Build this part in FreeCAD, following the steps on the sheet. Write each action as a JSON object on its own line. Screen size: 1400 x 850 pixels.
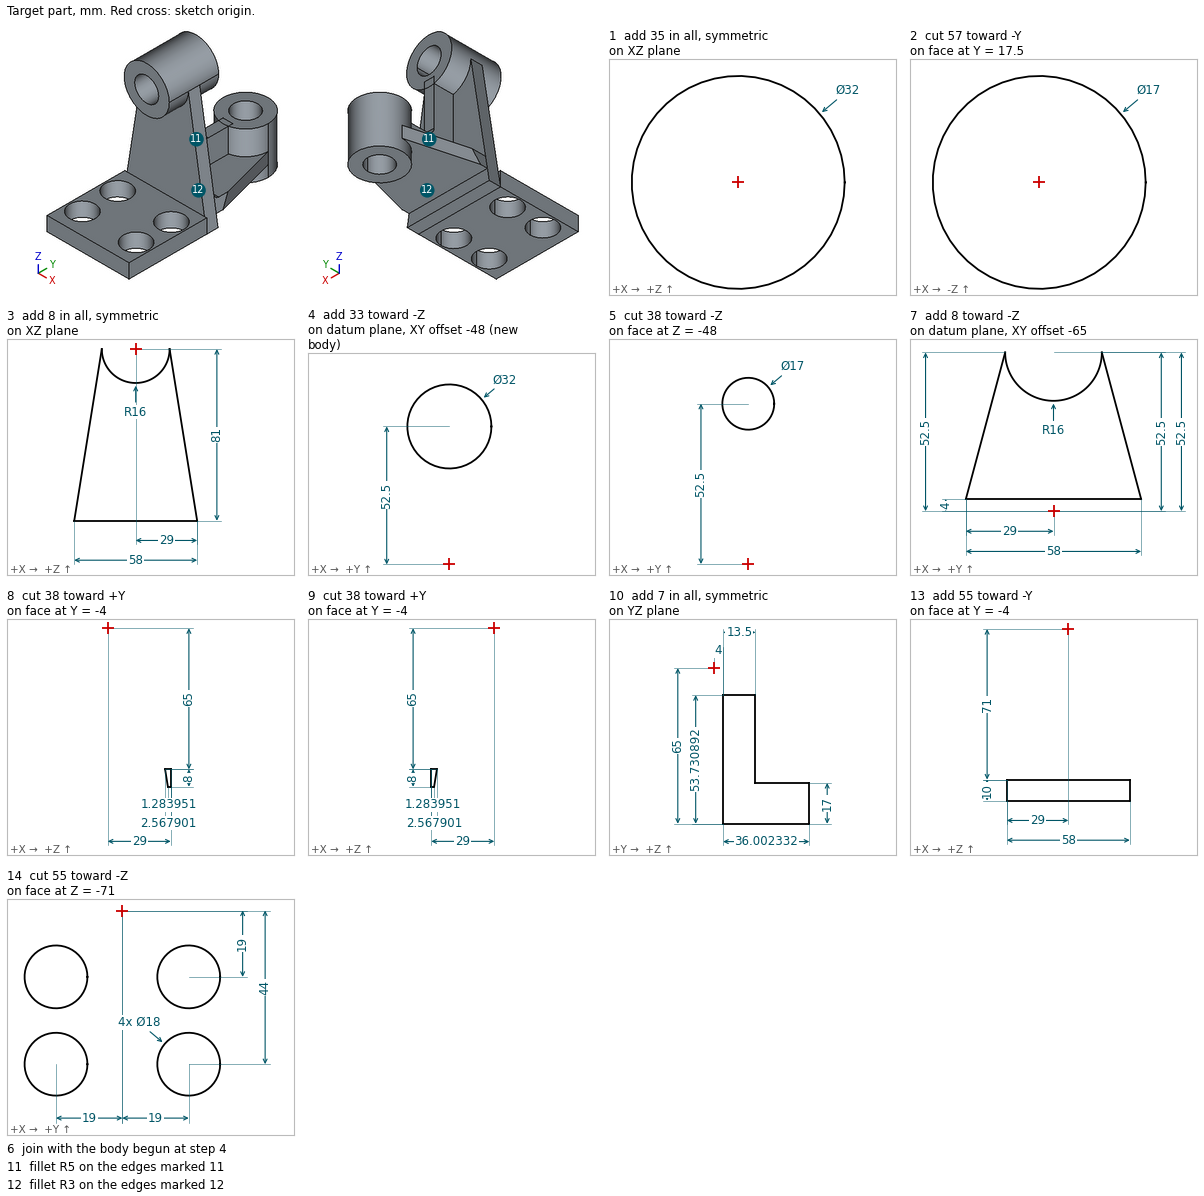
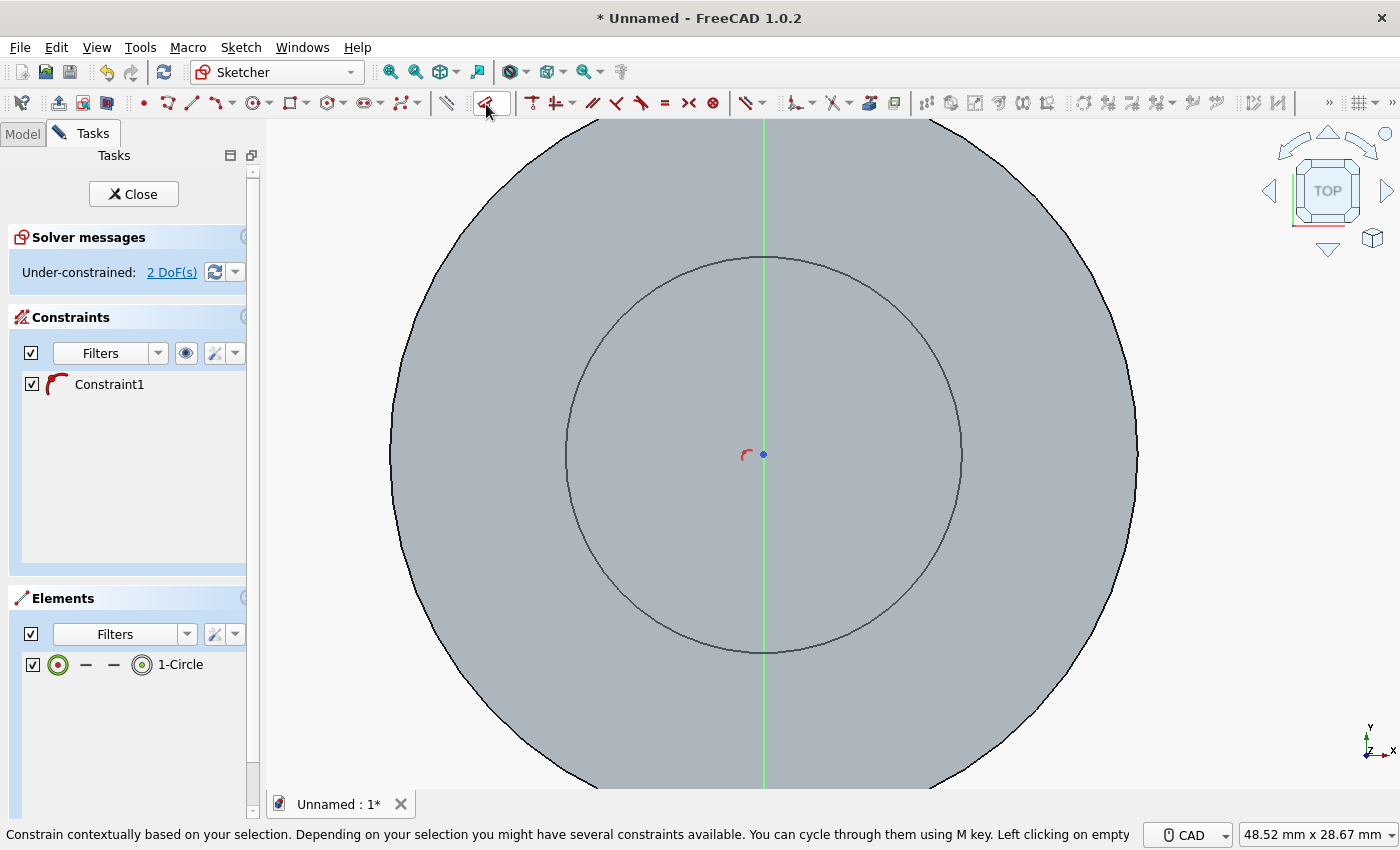
{"action": "left_click", "coordinate": [903, 314]}
{"action": "left_click", "coordinate": [925, 291]}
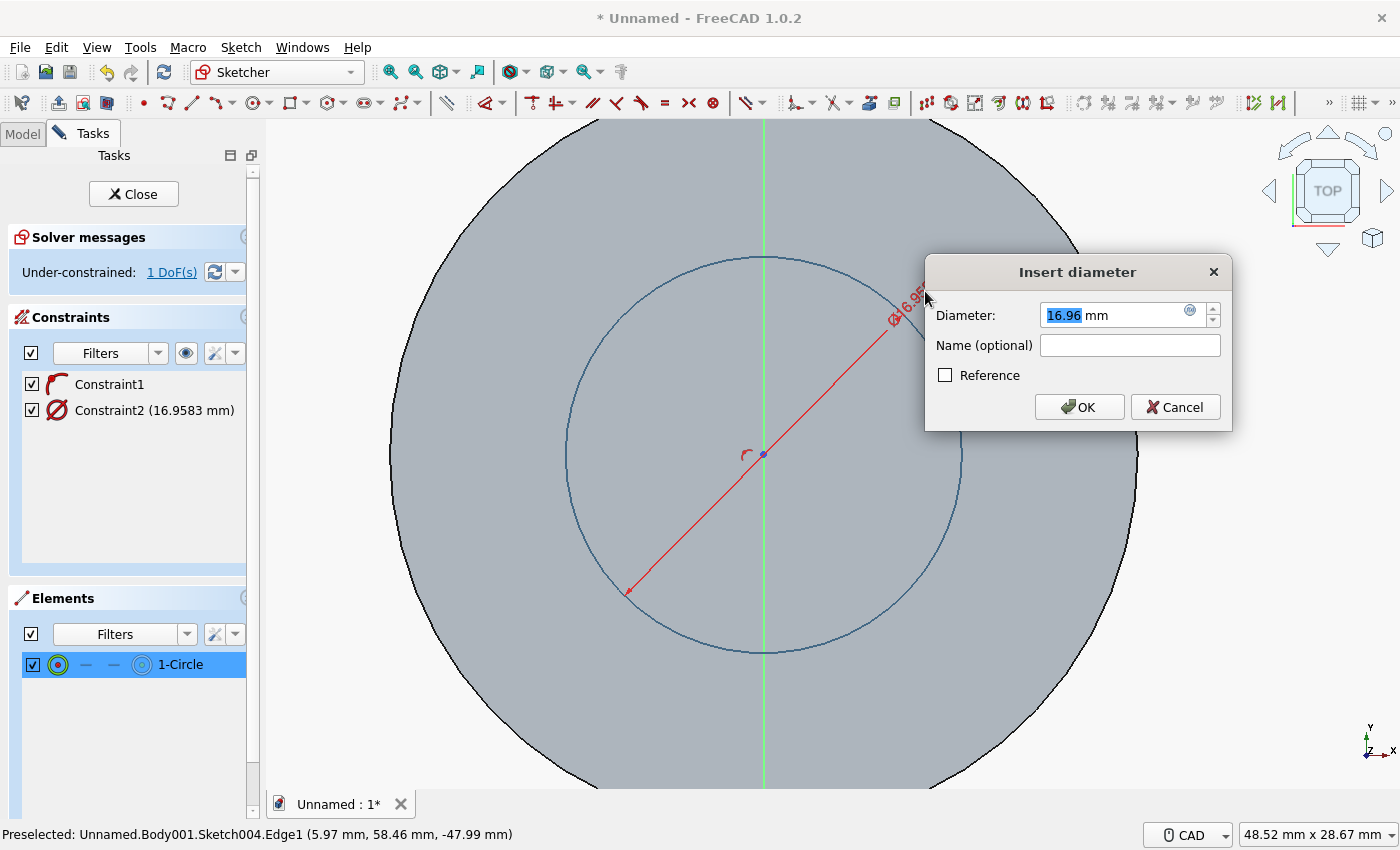
{"action": "type", "text": "17"}
{"action": "key", "text": "Return"}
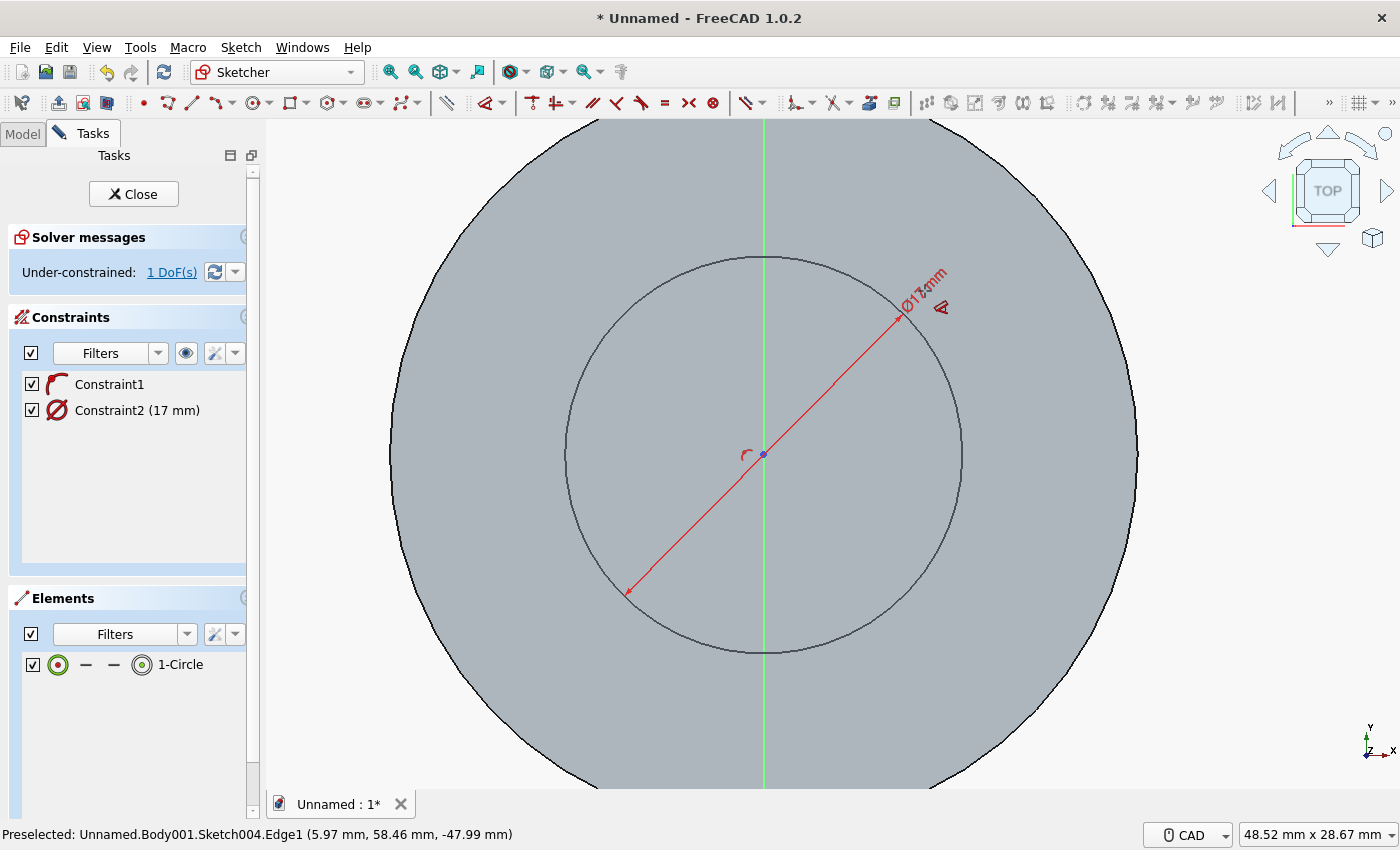
{"action": "left_click", "coordinate": [764, 455]}
{"action": "left_click", "coordinate": [798, 608]}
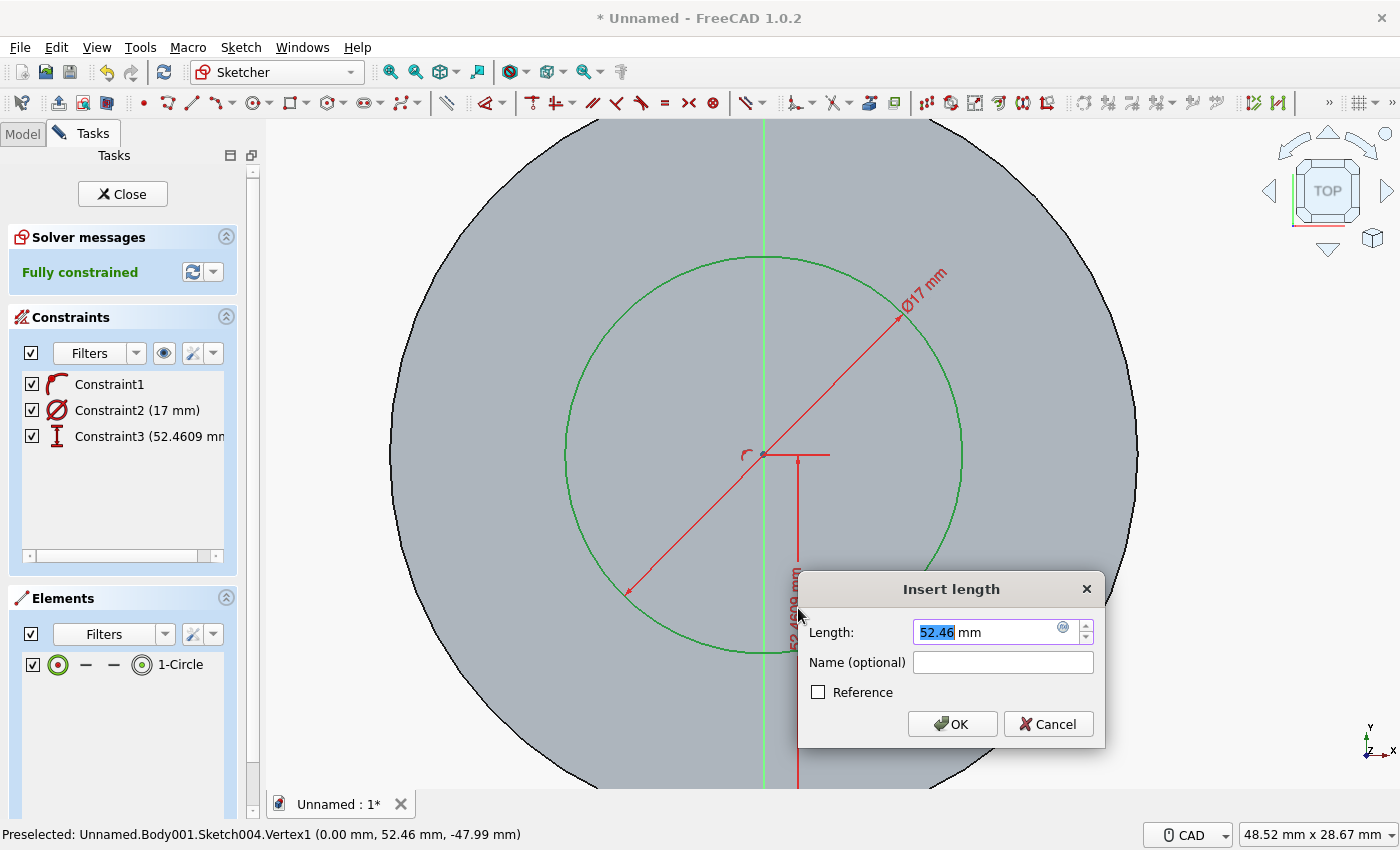
{"action": "type", "text": "52.5"}
{"action": "key", "text": "Return"}
{"action": "key", "text": "Escape"}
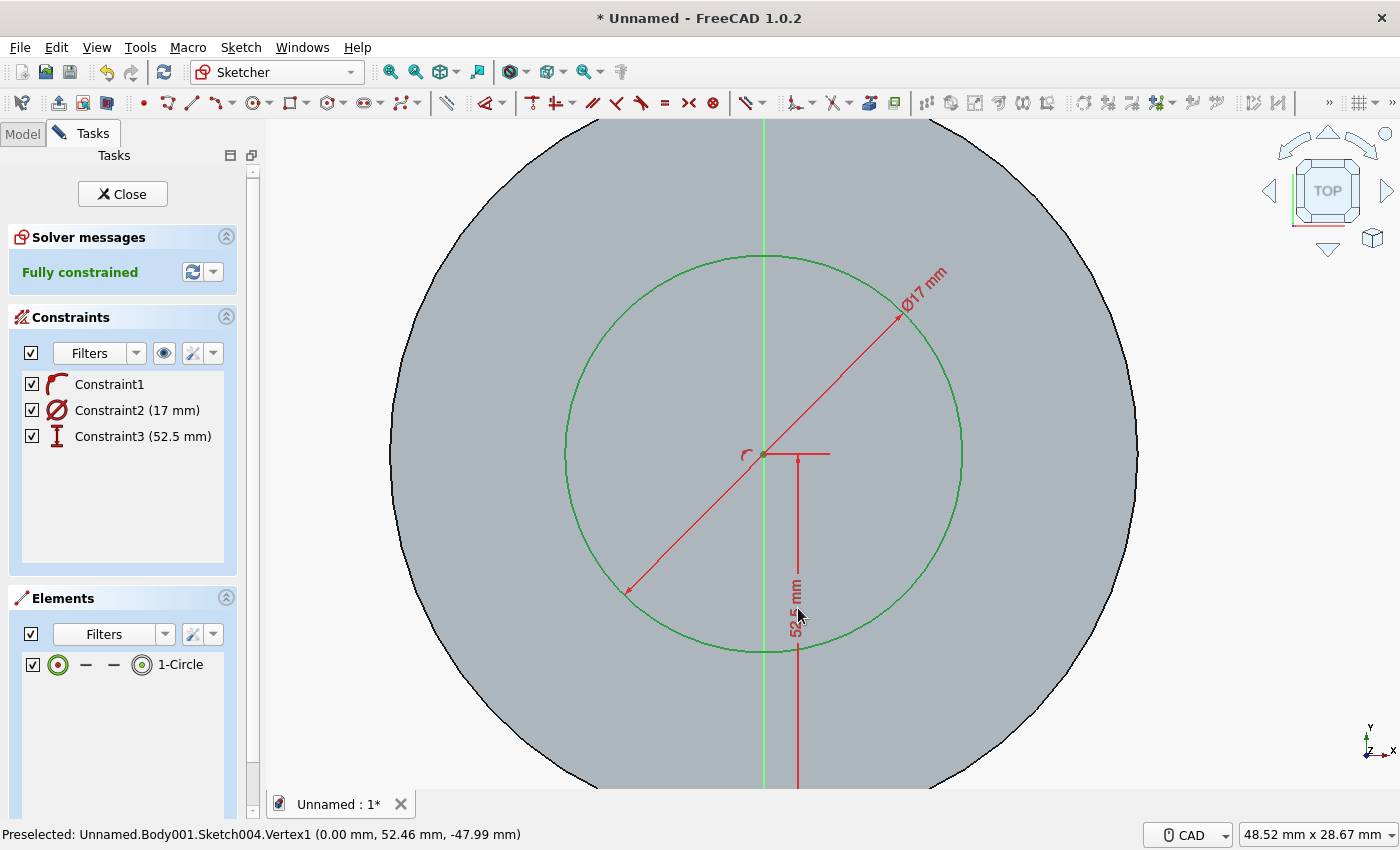
{"action": "left_click", "coordinate": [123, 194]}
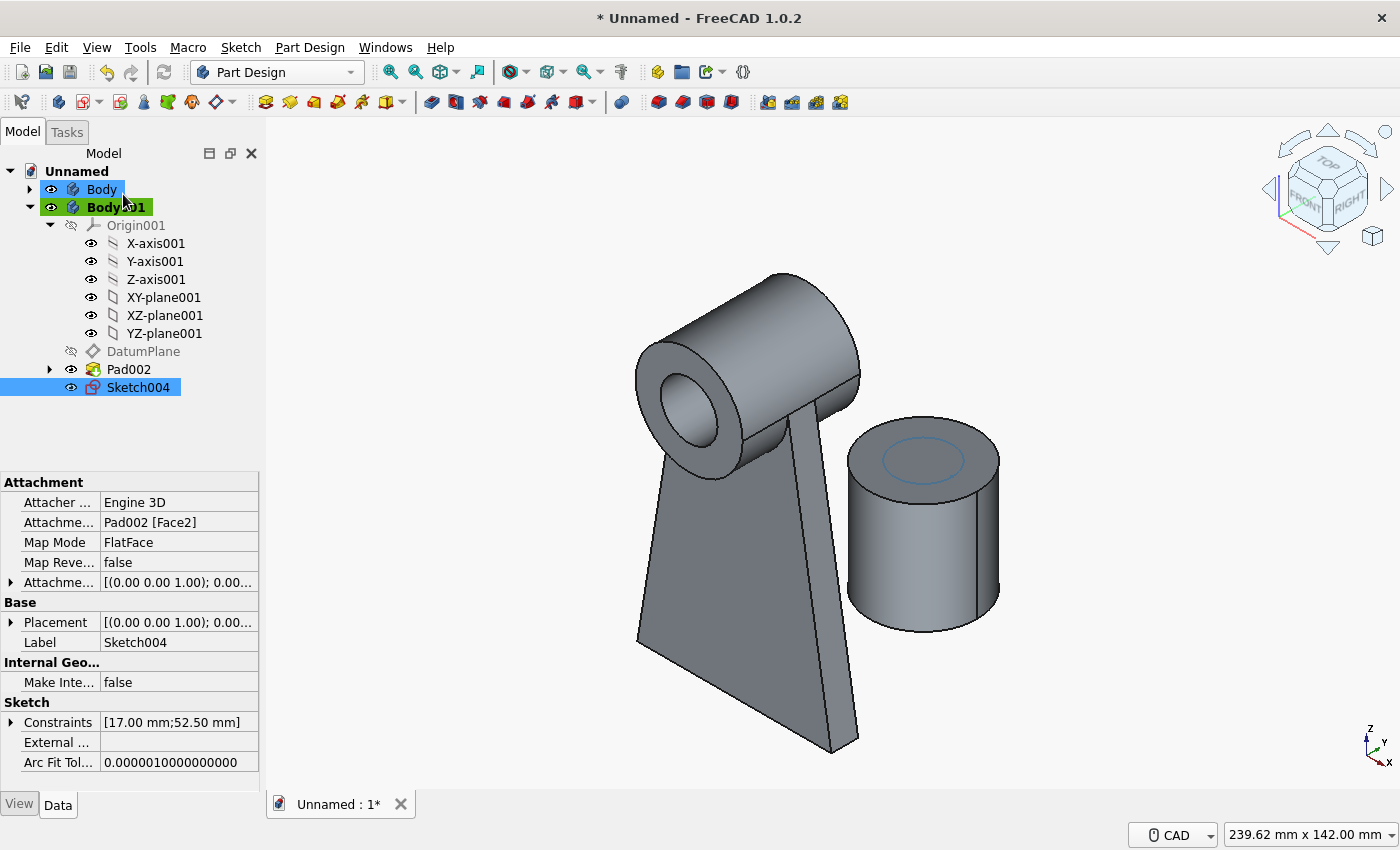
{"action": "left_click", "coordinate": [432, 102]}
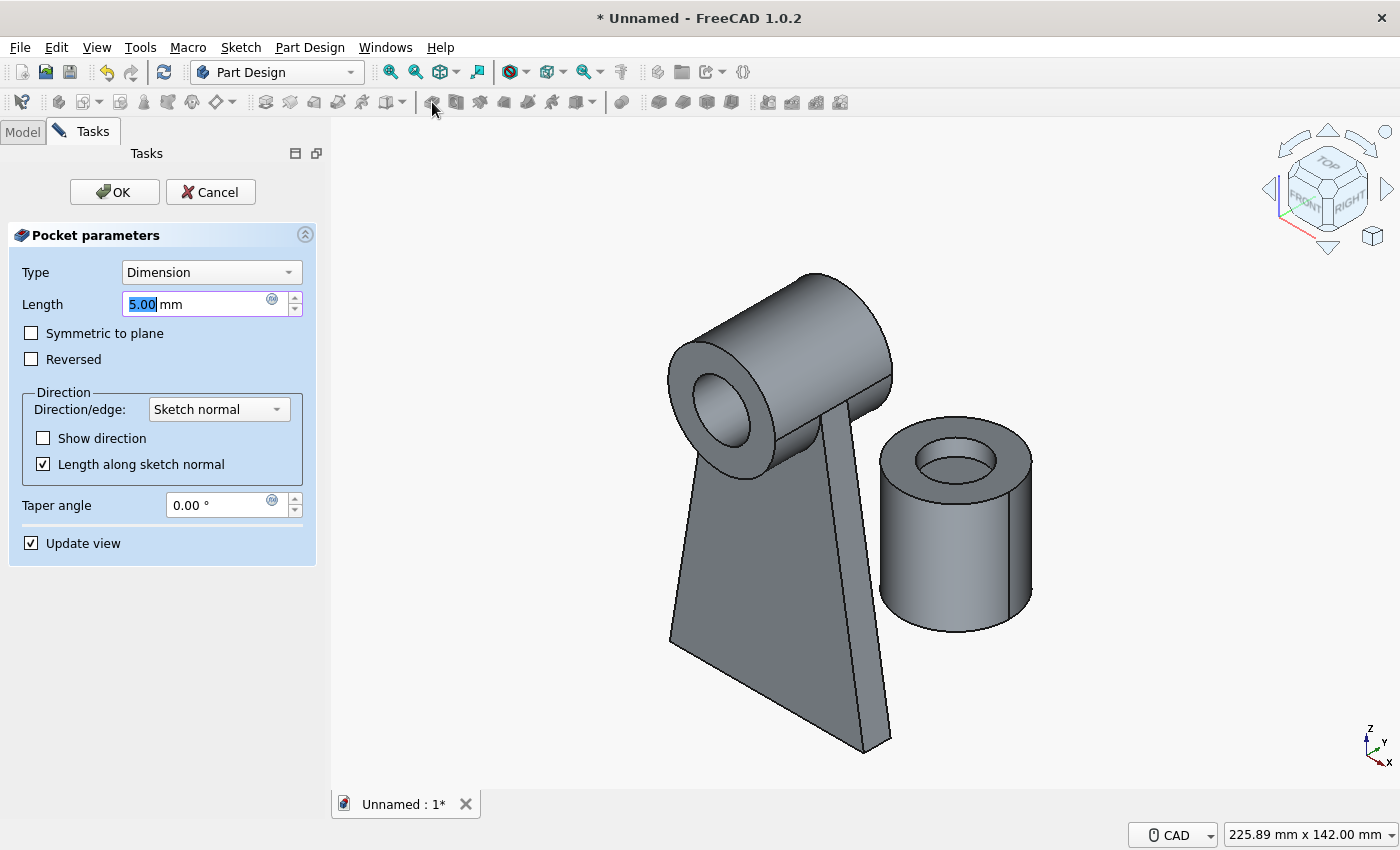
{"action": "type", "text": "38"}
{"action": "key", "text": "Tab"}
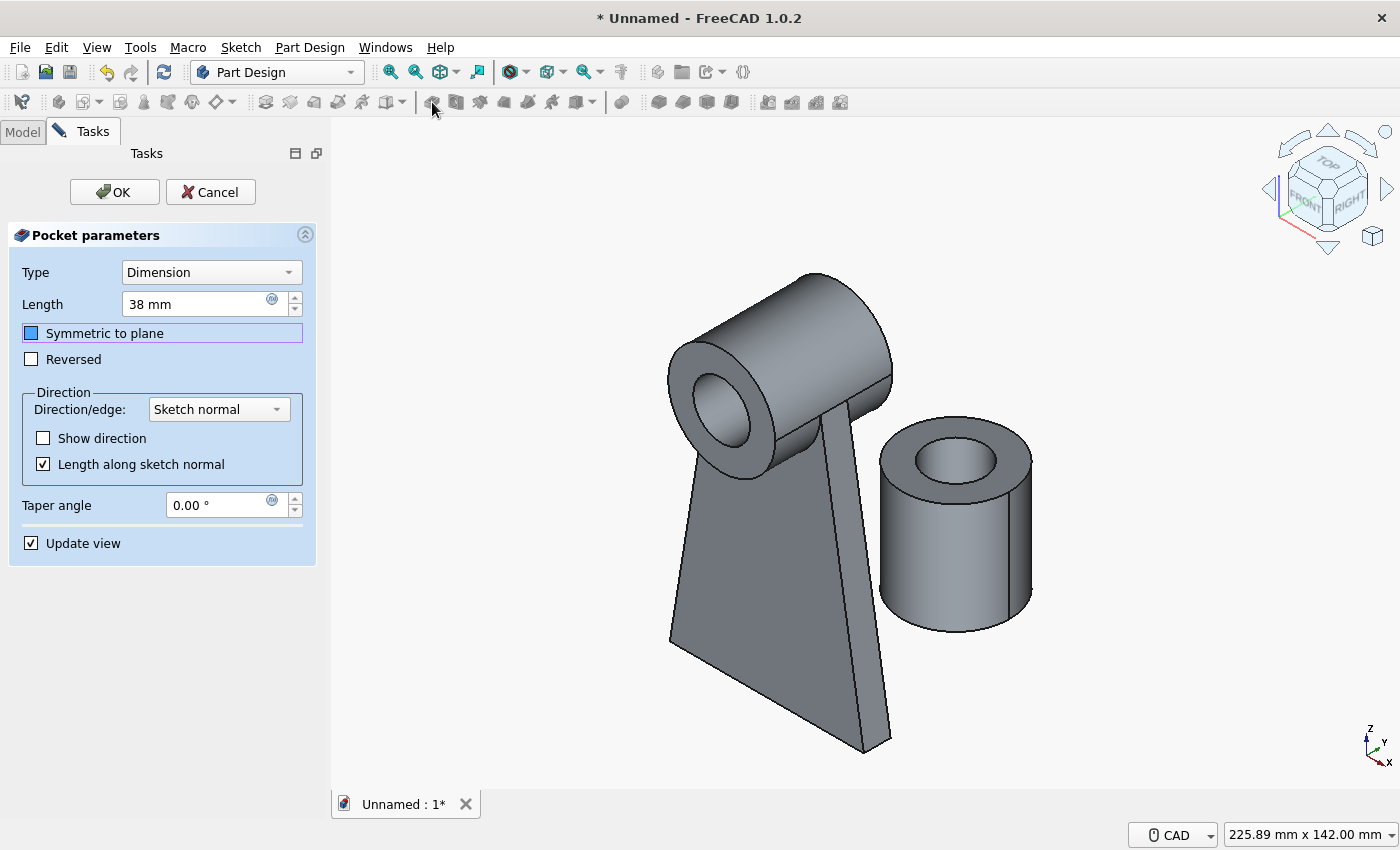
{"action": "left_click", "coordinate": [115, 192]}